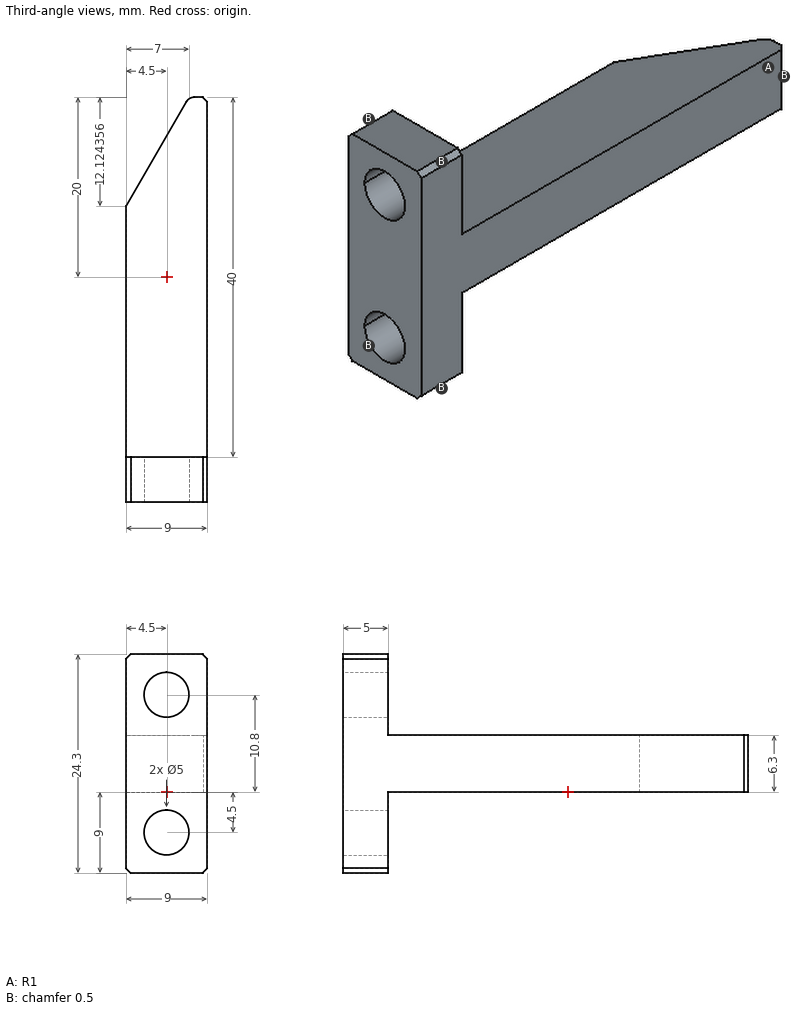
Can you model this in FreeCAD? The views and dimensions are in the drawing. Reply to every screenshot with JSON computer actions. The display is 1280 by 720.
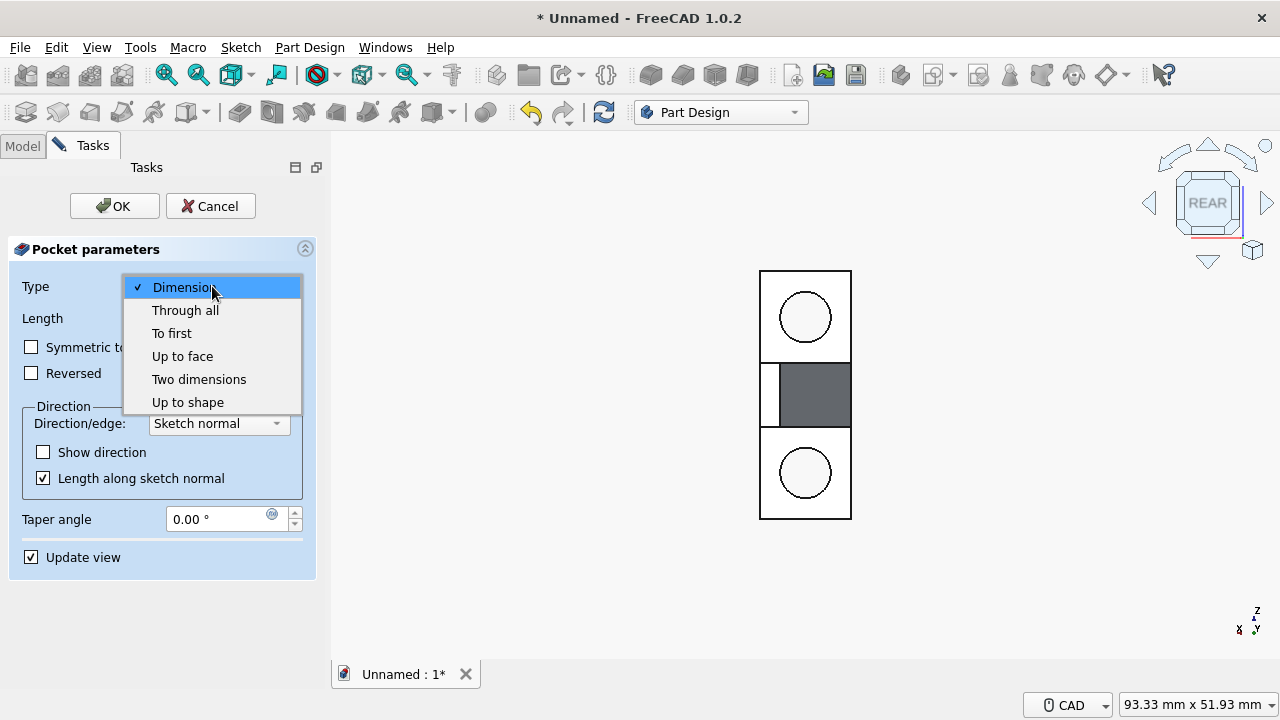
{"action": "left_click", "coordinate": [212, 310]}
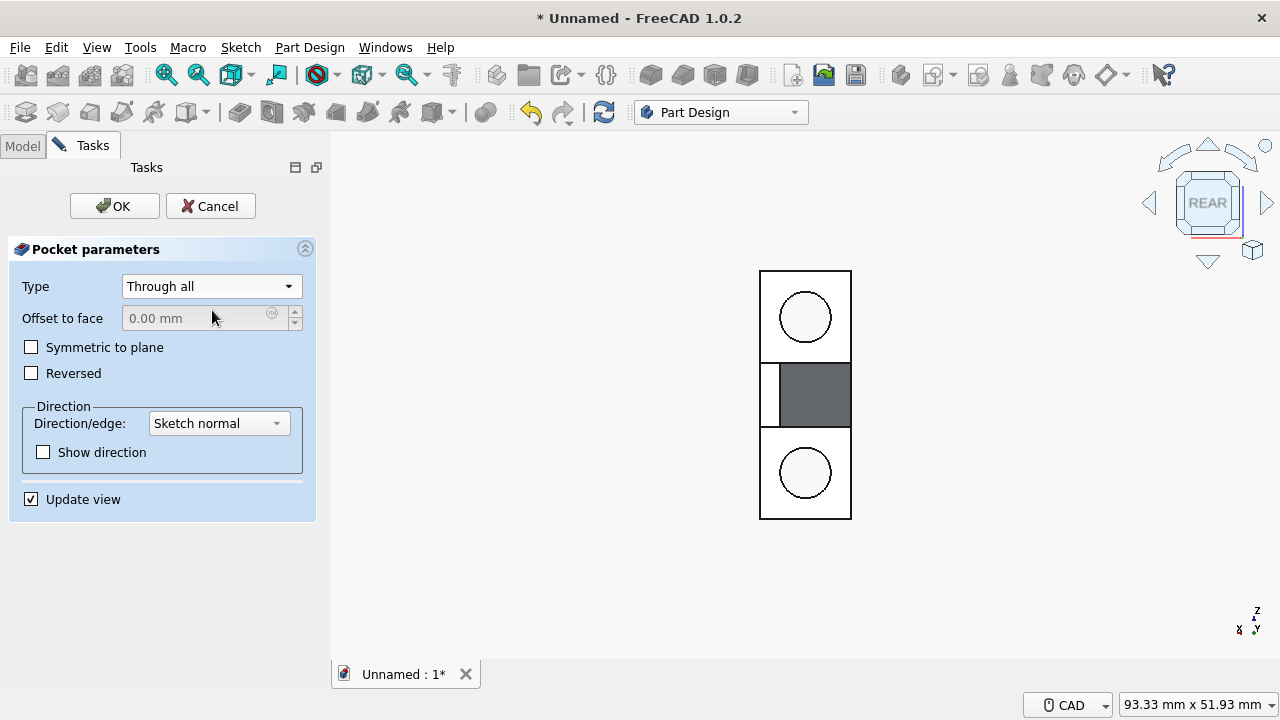
{"action": "left_click", "coordinate": [115, 206]}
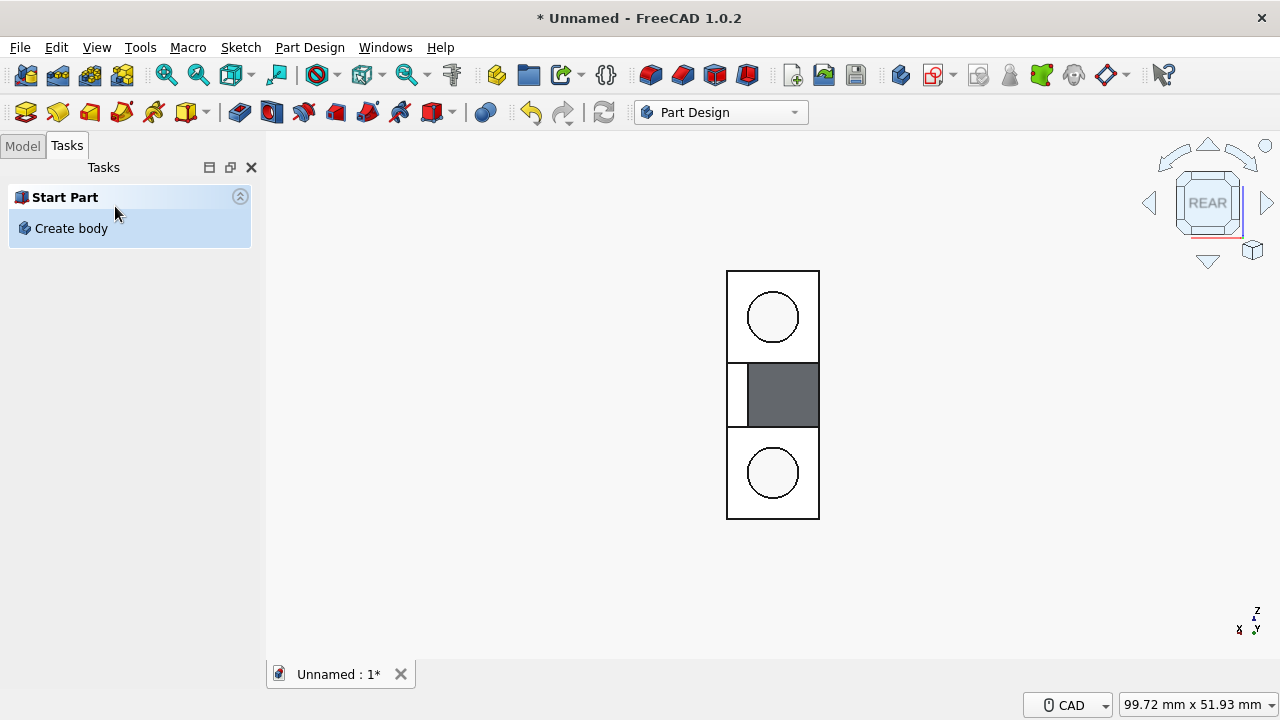
{"action": "left_click", "coordinate": [748, 394]}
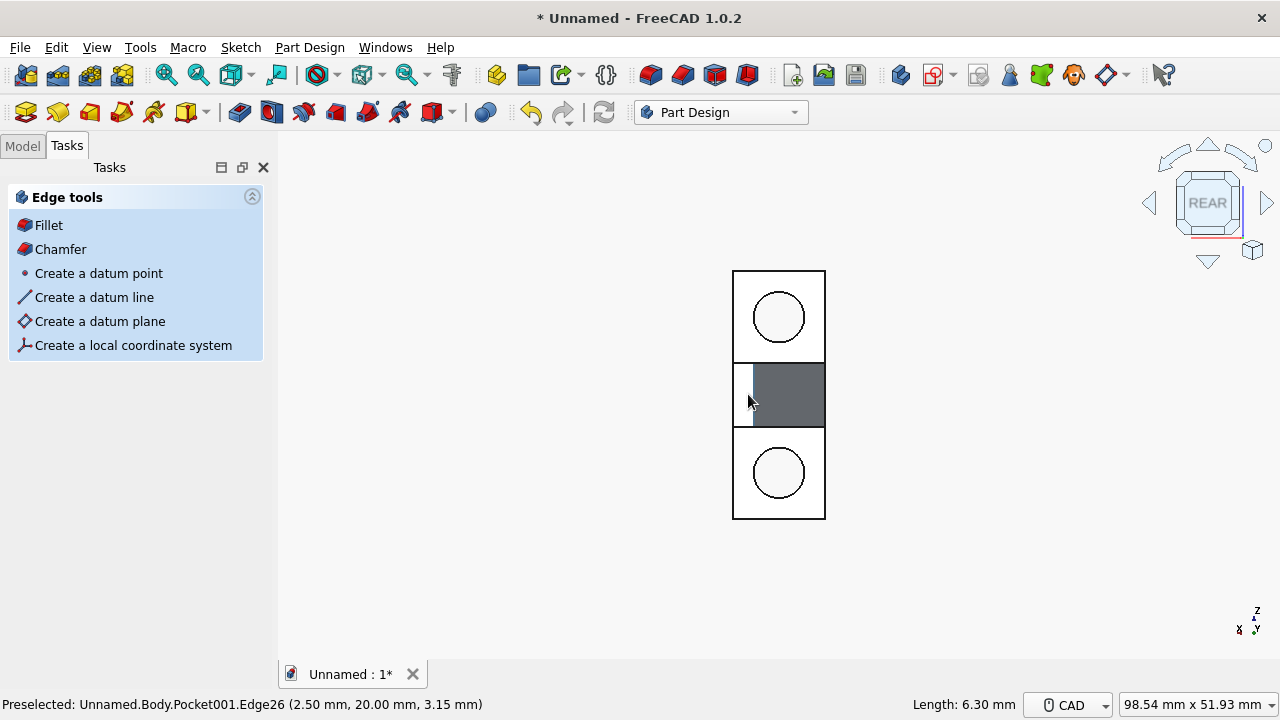
{"action": "left_click", "coordinate": [652, 76]}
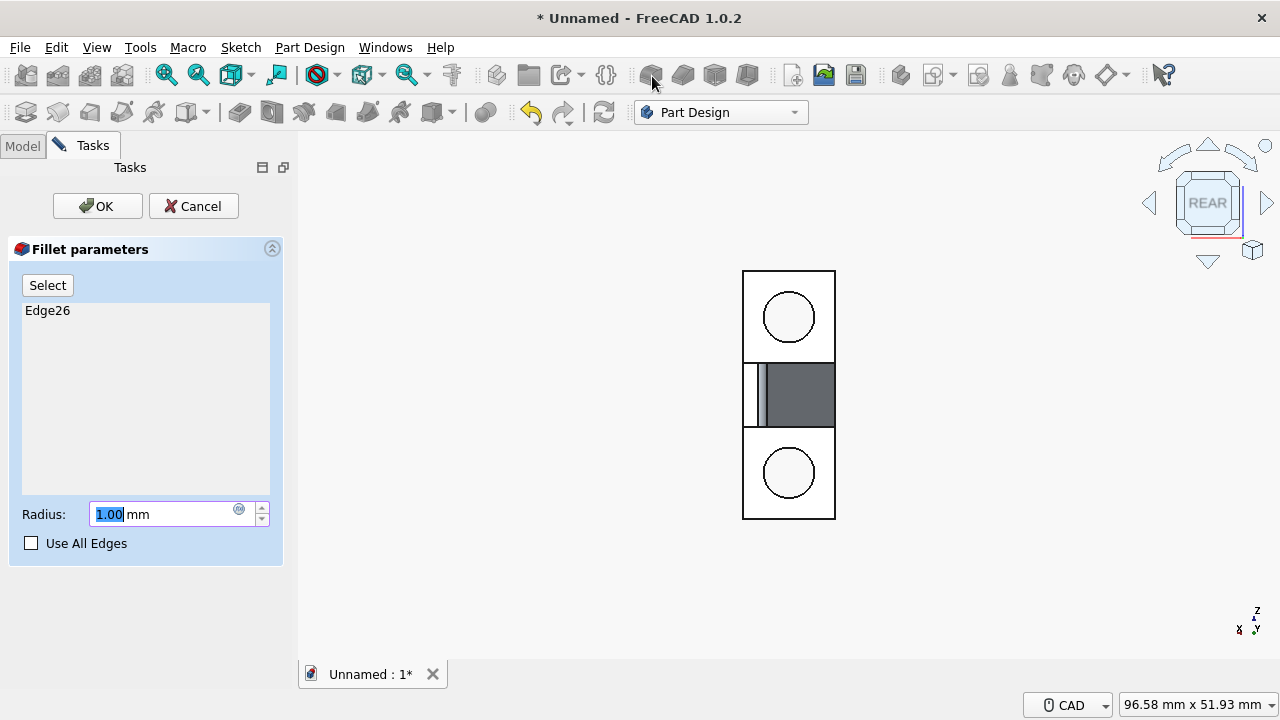
{"action": "type", "text": "1"}
{"action": "key", "text": "Tab"}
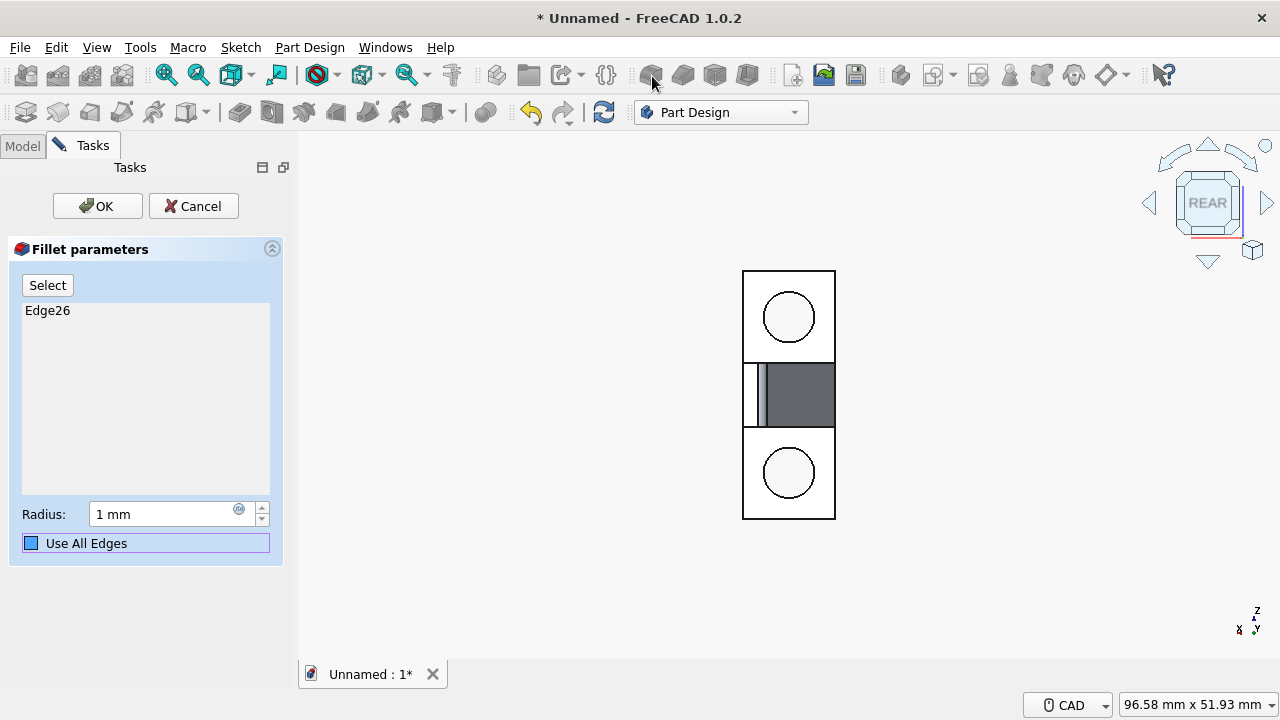
{"action": "left_click", "coordinate": [98, 206]}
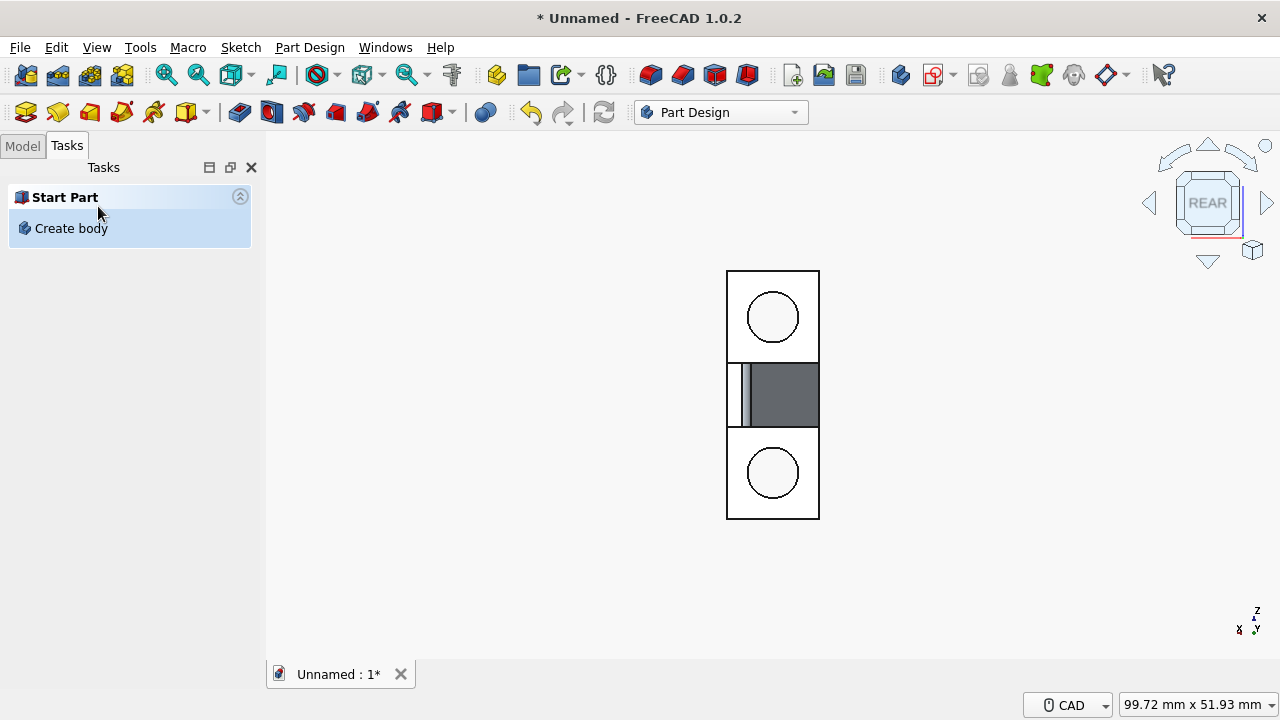
{"action": "key", "text": "0"}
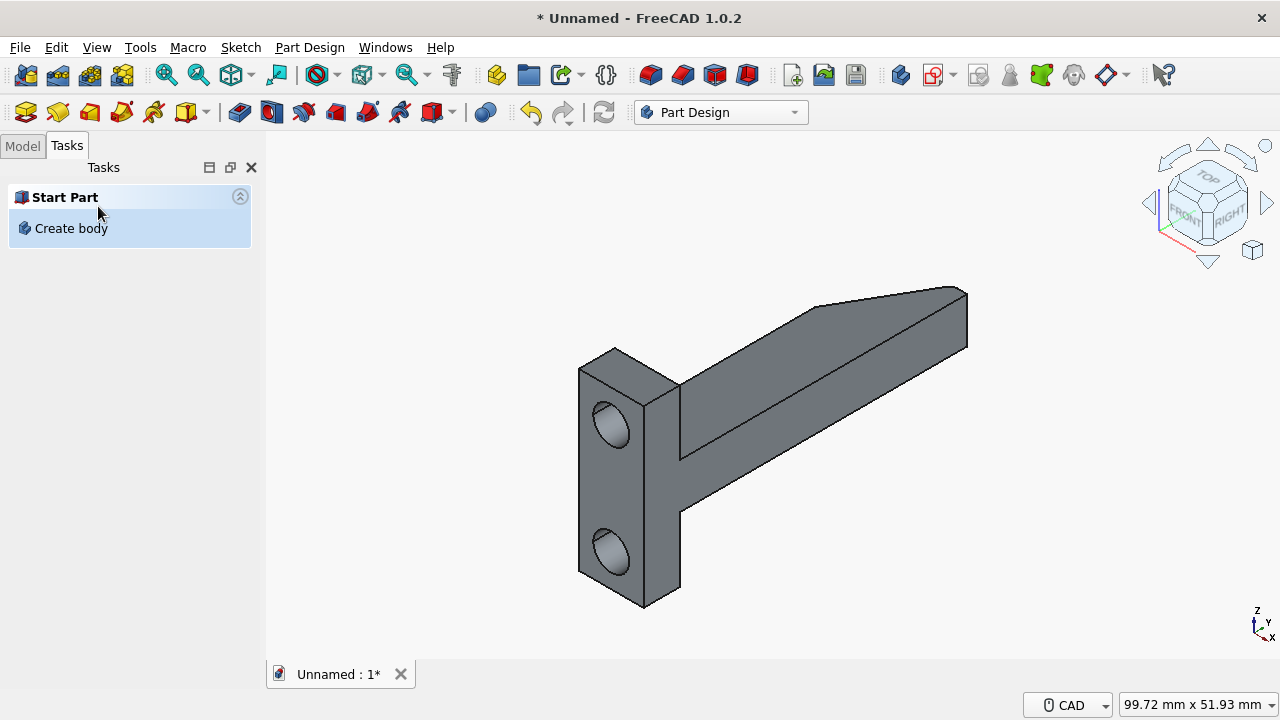
{"action": "left_click", "coordinate": [662, 395]}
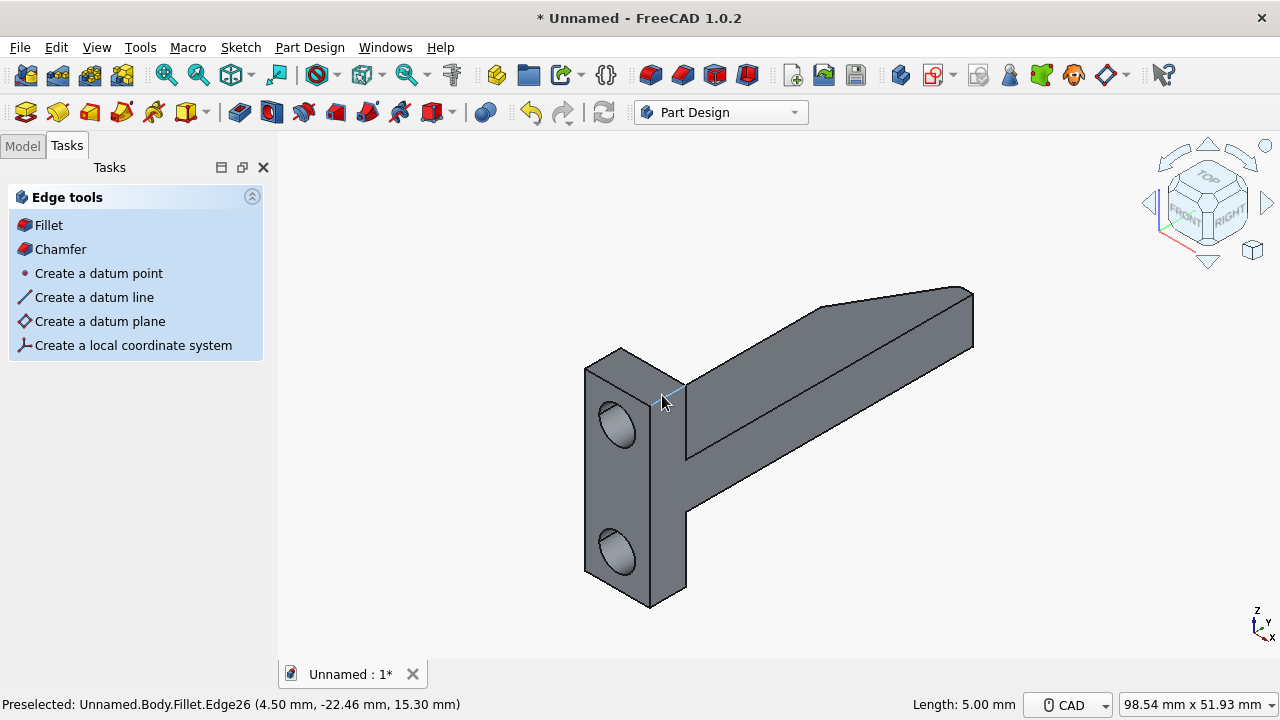
{"action": "key", "text": "2"}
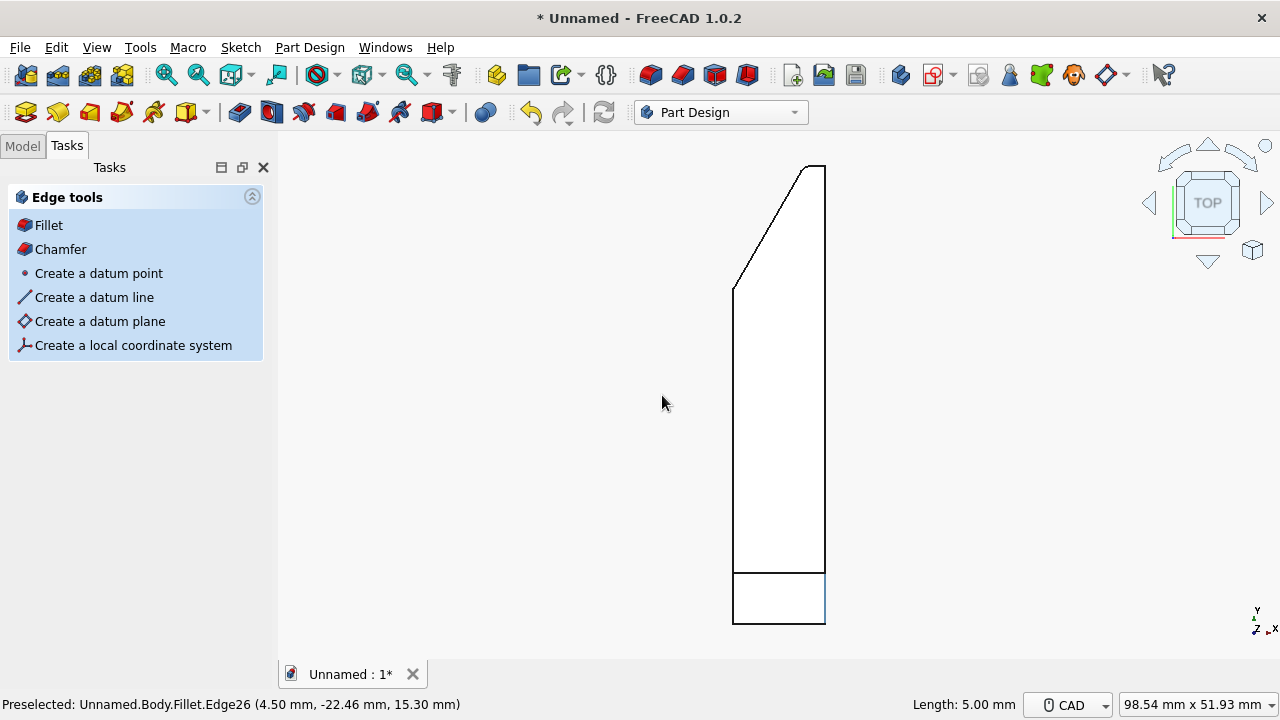
{"action": "left_click", "coordinate": [733, 597], "text": "ctrl"}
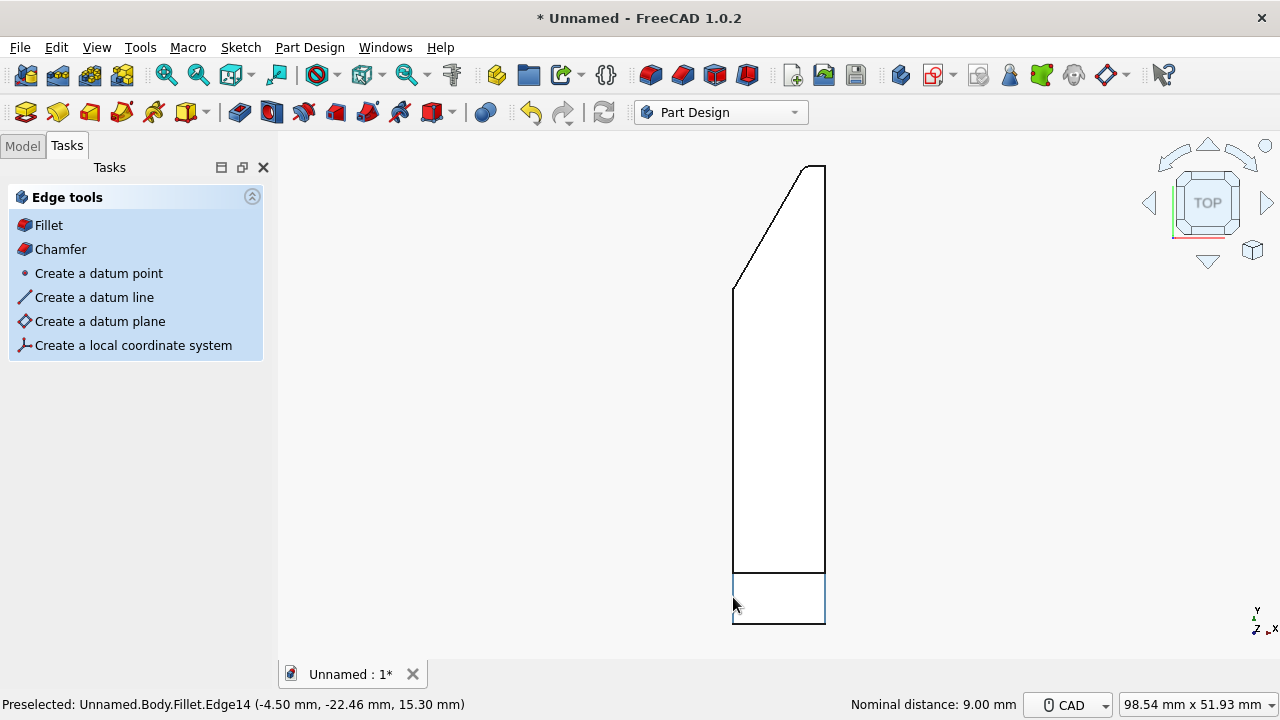
{"action": "key", "text": "1"}